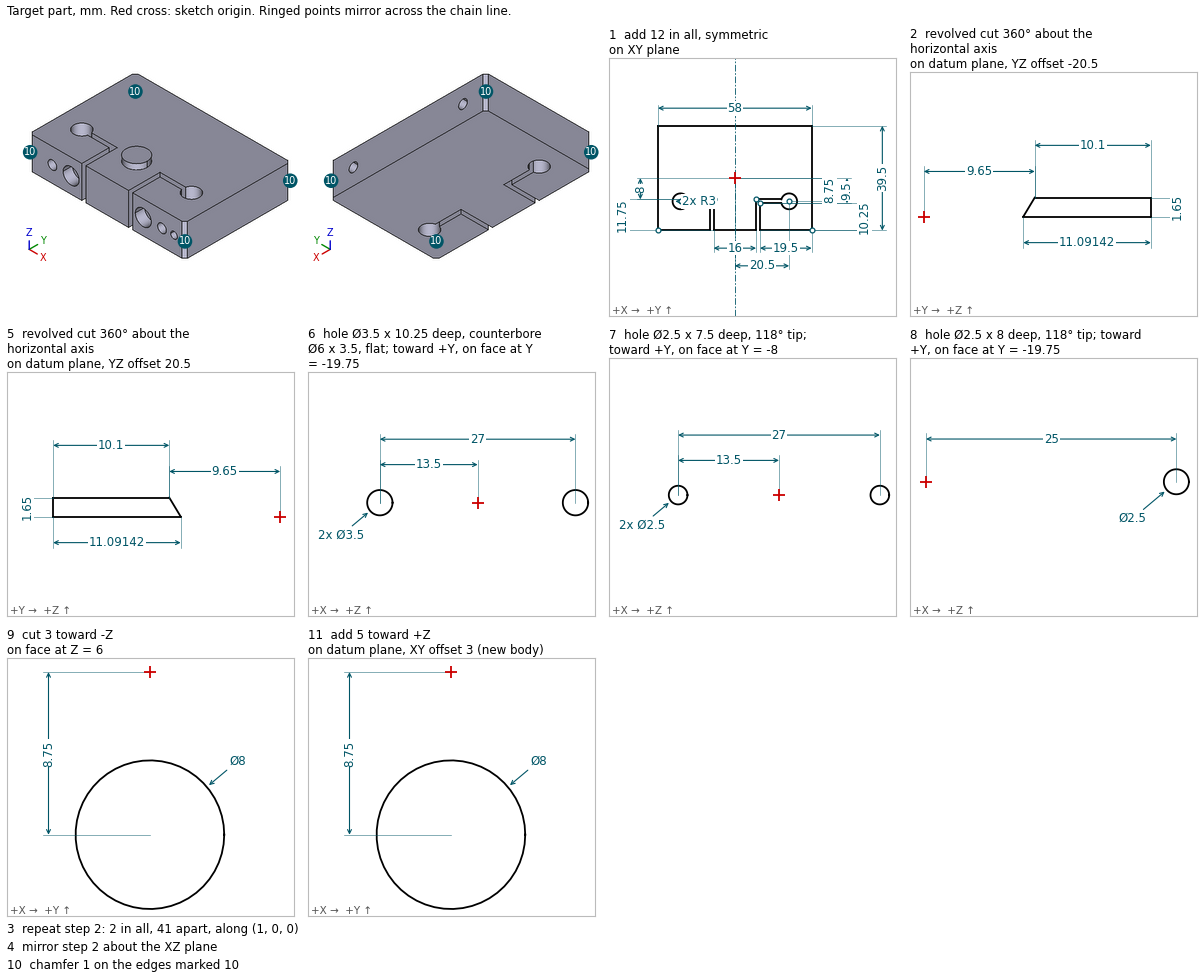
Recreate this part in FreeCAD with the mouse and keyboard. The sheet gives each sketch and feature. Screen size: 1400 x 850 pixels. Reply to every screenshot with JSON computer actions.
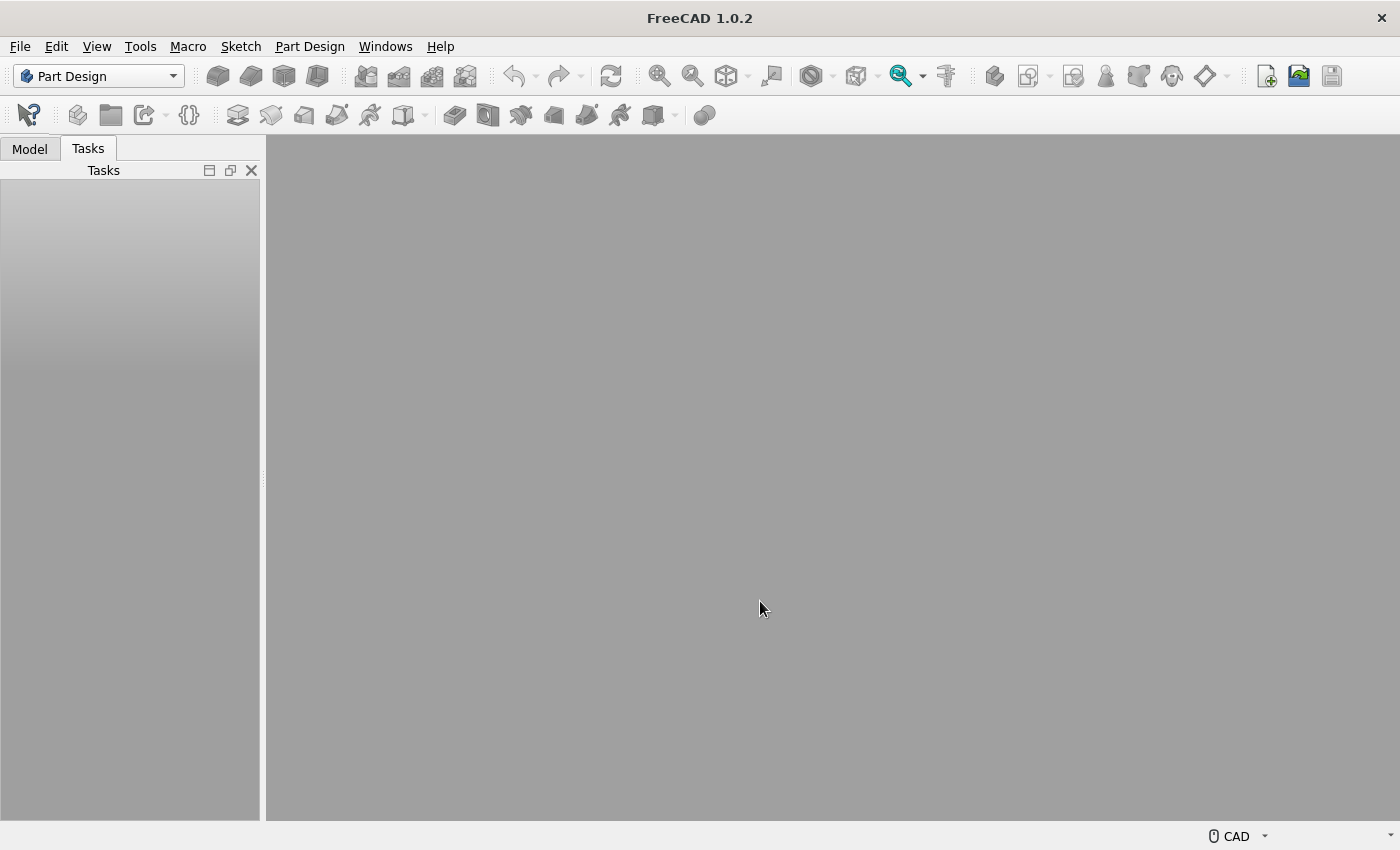
{"action": "left_click", "coordinate": [1266, 76]}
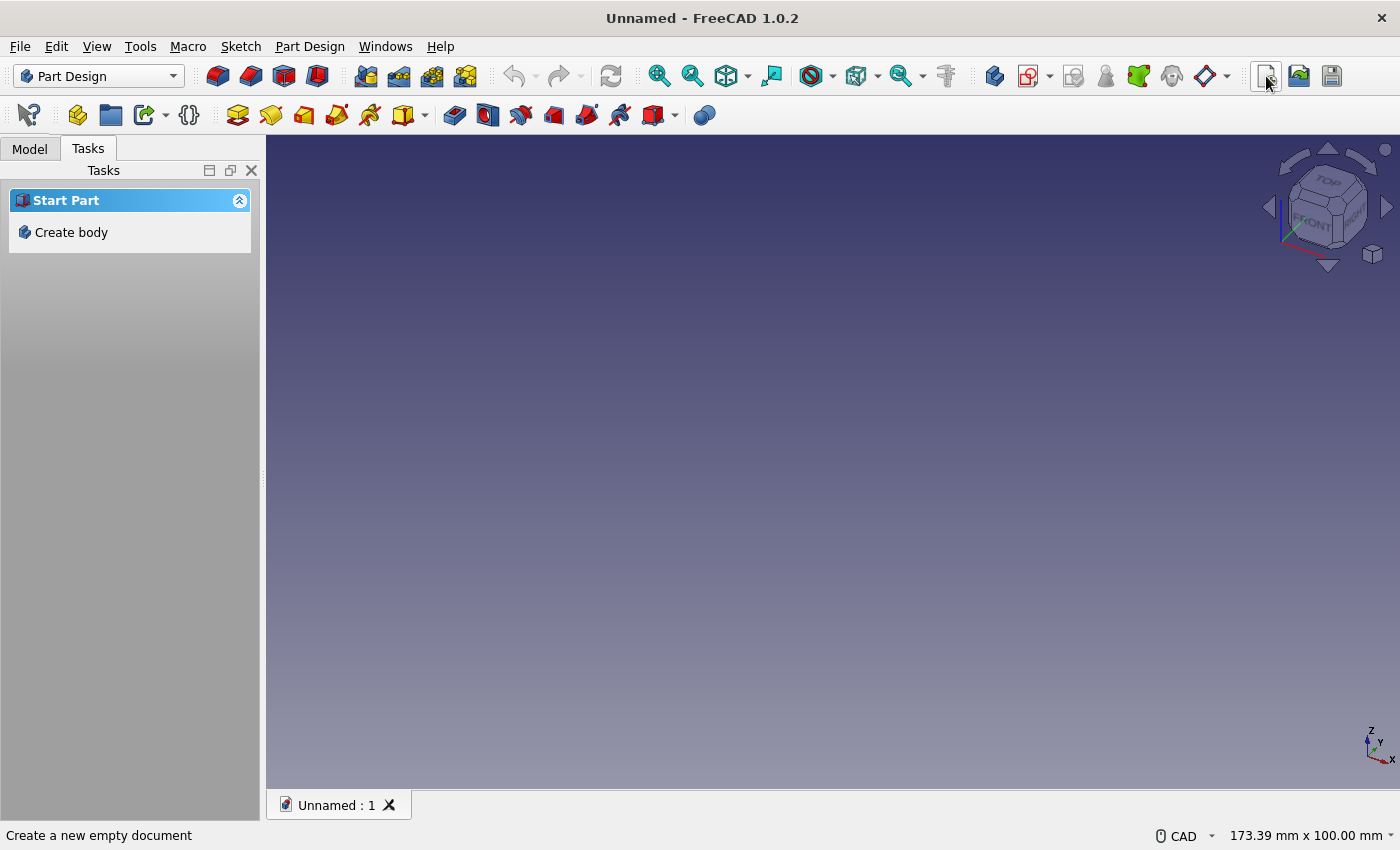
{"action": "left_click", "coordinate": [1028, 76]}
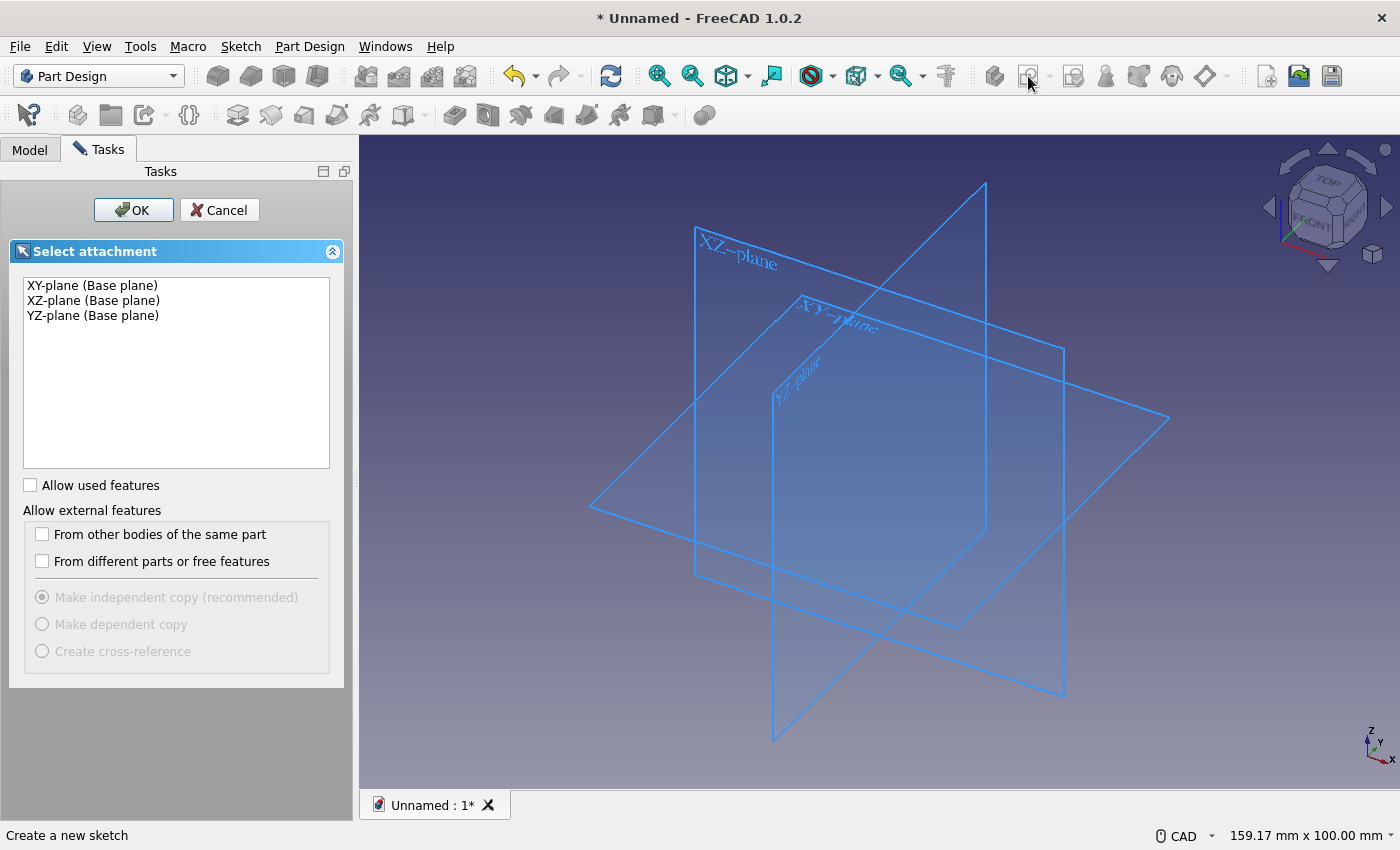
{"action": "left_click", "coordinate": [84, 286]}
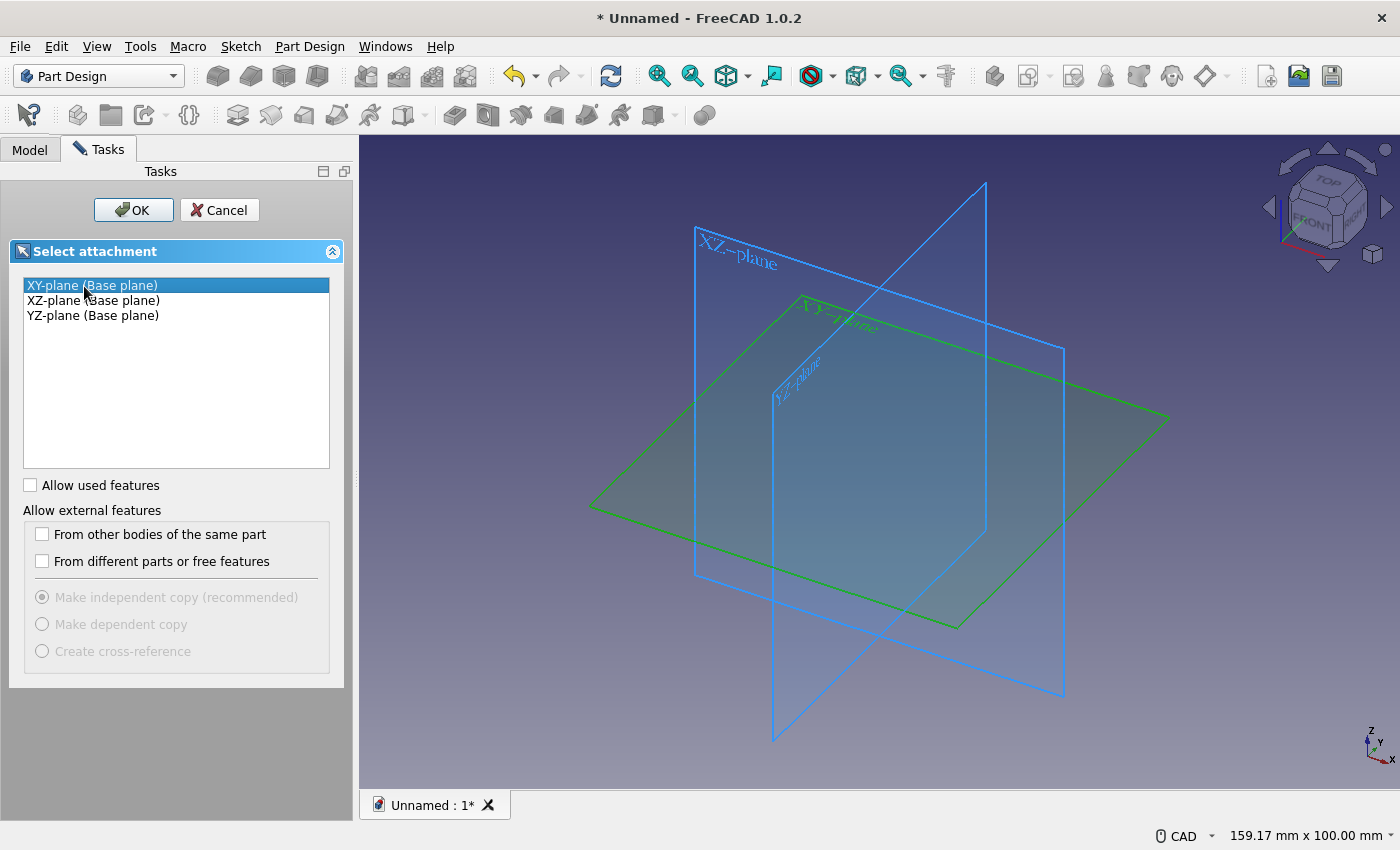
{"action": "left_click", "coordinate": [134, 210]}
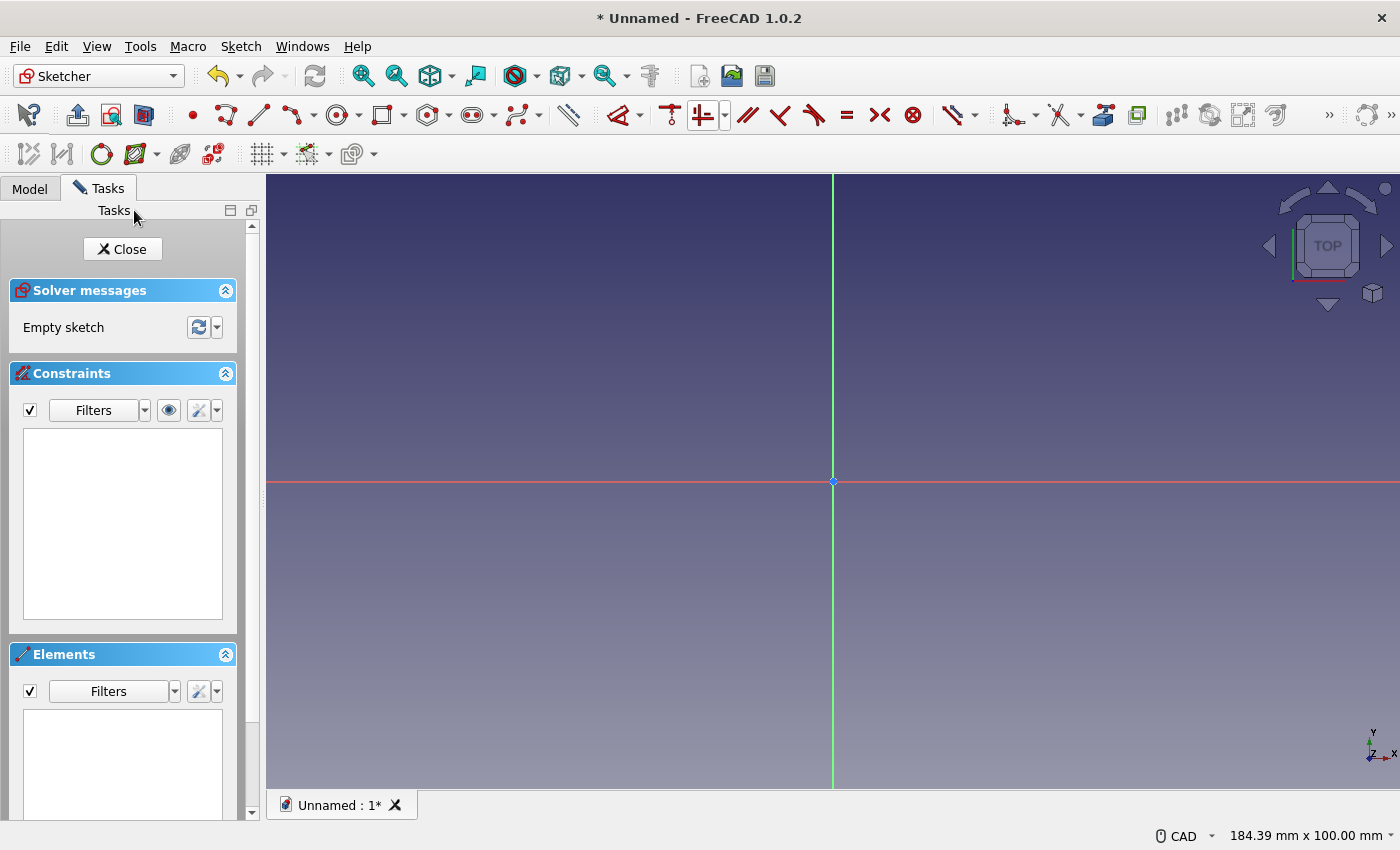
{"action": "scroll", "coordinate": [972, 482], "scroll_direction": "up", "scroll_amount": 2}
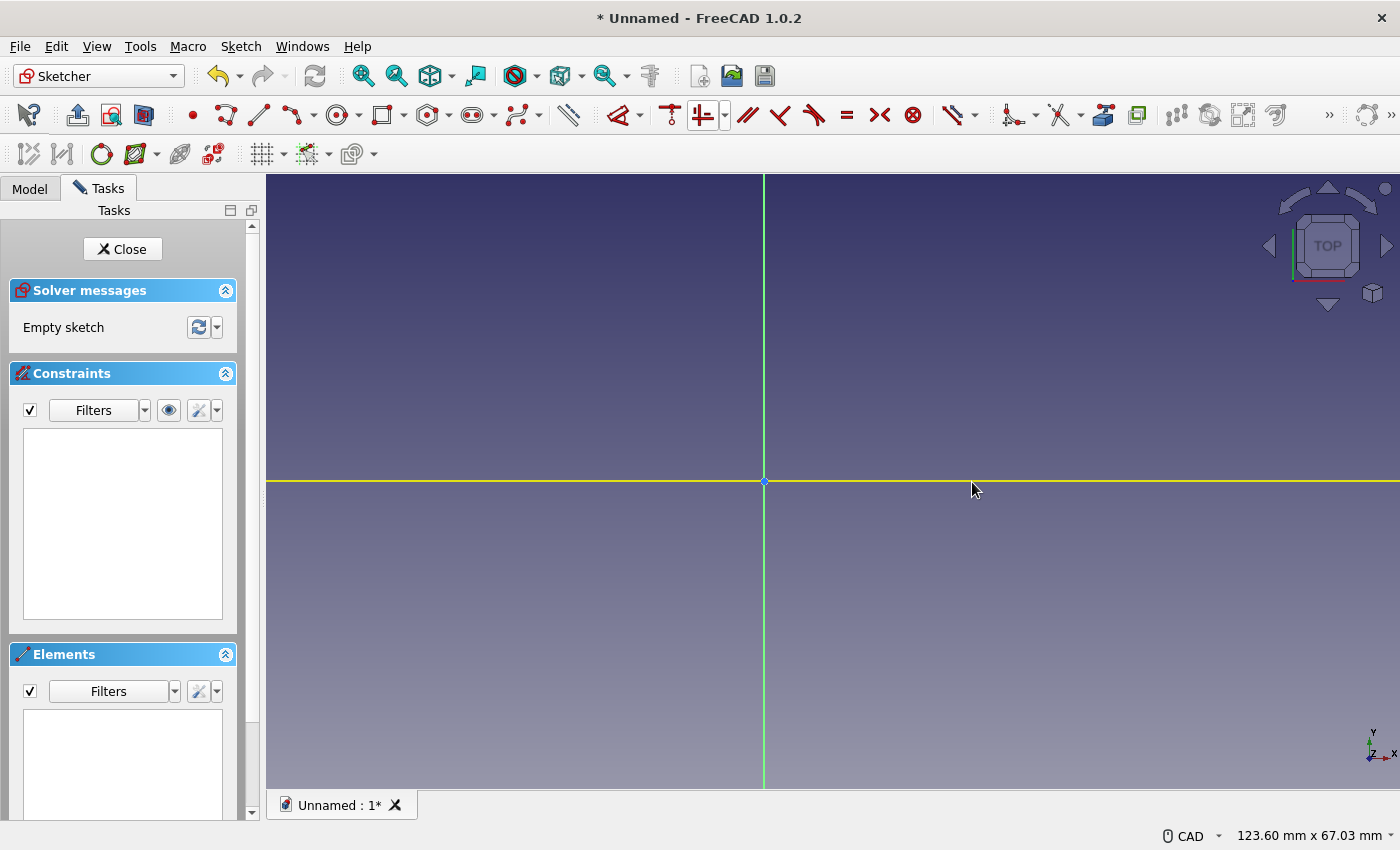
{"action": "left_click", "coordinate": [226, 116]}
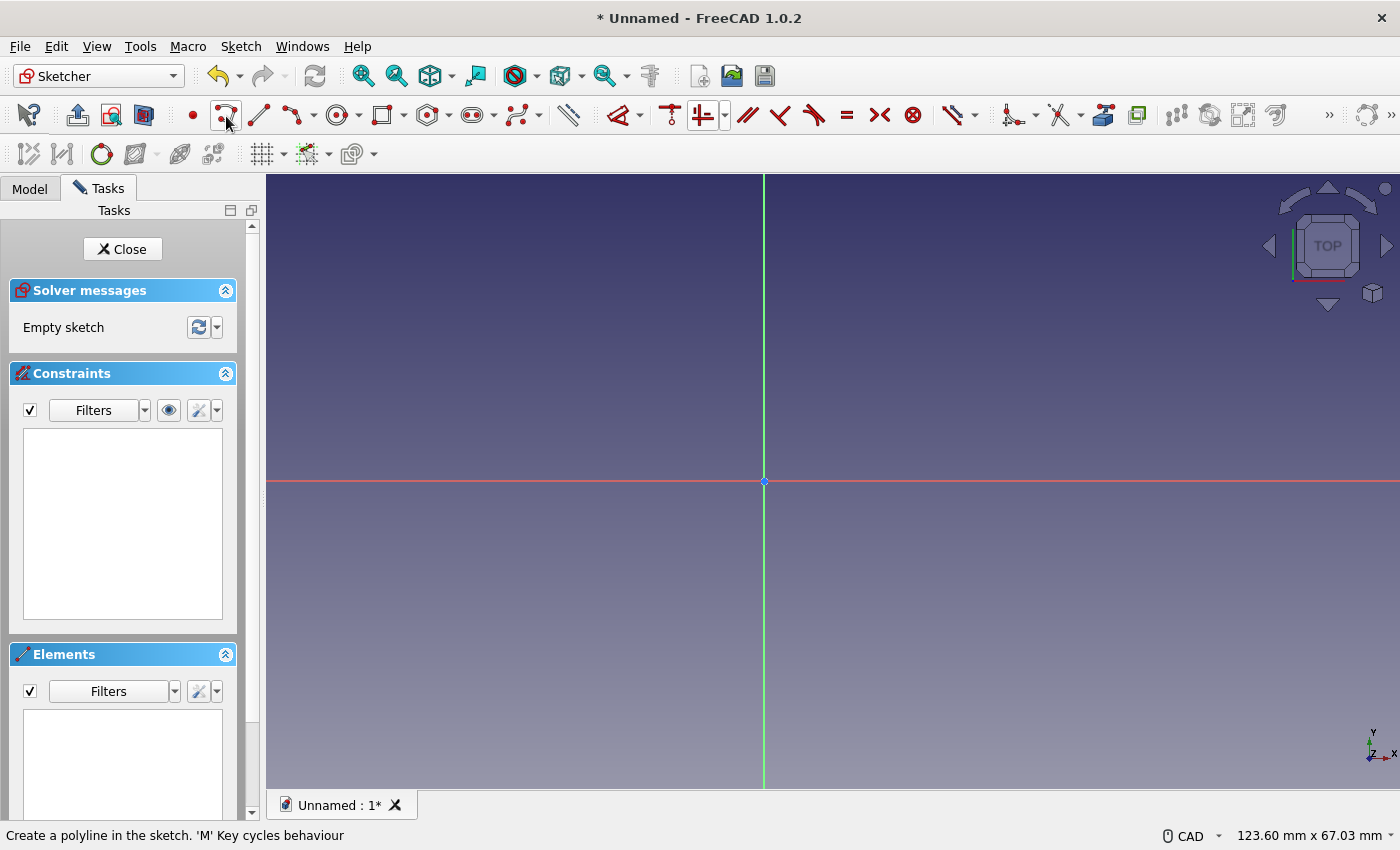
{"action": "left_click", "coordinate": [603, 554]}
{"action": "left_click", "coordinate": [691, 554]}
{"action": "left_click", "coordinate": [691, 662]}
{"action": "left_click", "coordinate": [838, 662]}
{"action": "left_click", "coordinate": [838, 554]}
{"action": "left_click", "coordinate": [926, 554]}
{"action": "right_click", "coordinate": [926, 554]}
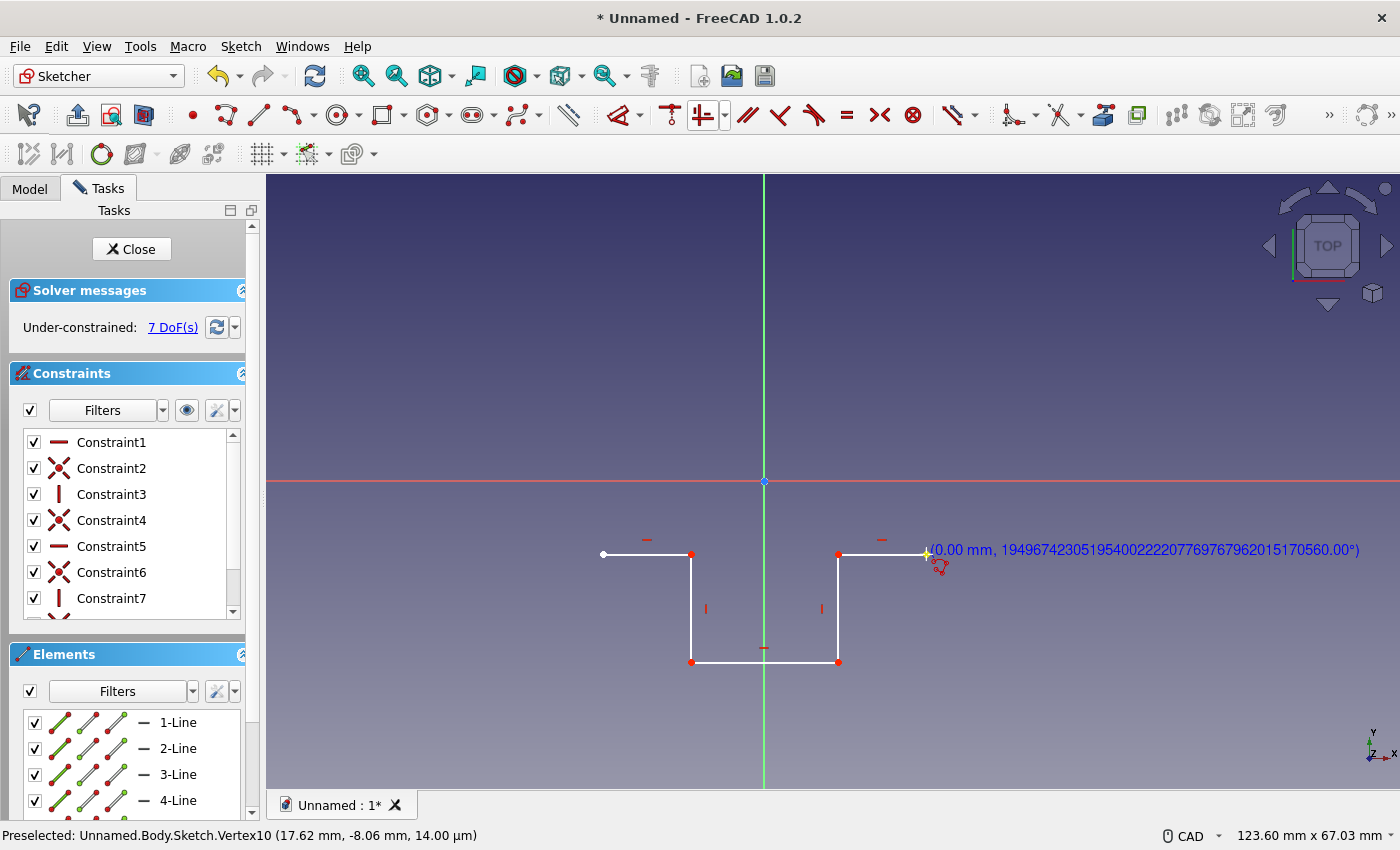
{"action": "left_click", "coordinate": [926, 568]}
{"action": "left_click", "coordinate": [851, 568]}
{"action": "left_click", "coordinate": [851, 662]}
{"action": "left_click", "coordinate": [1030, 662]}
{"action": "left_click", "coordinate": [1030, 300]}
{"action": "left_click", "coordinate": [498, 300]}
{"action": "left_click", "coordinate": [498, 662]}
{"action": "left_click", "coordinate": [677, 662]}
{"action": "left_click", "coordinate": [677, 568]}
{"action": "left_click", "coordinate": [603, 568]}
{"action": "right_click", "coordinate": [603, 568]}